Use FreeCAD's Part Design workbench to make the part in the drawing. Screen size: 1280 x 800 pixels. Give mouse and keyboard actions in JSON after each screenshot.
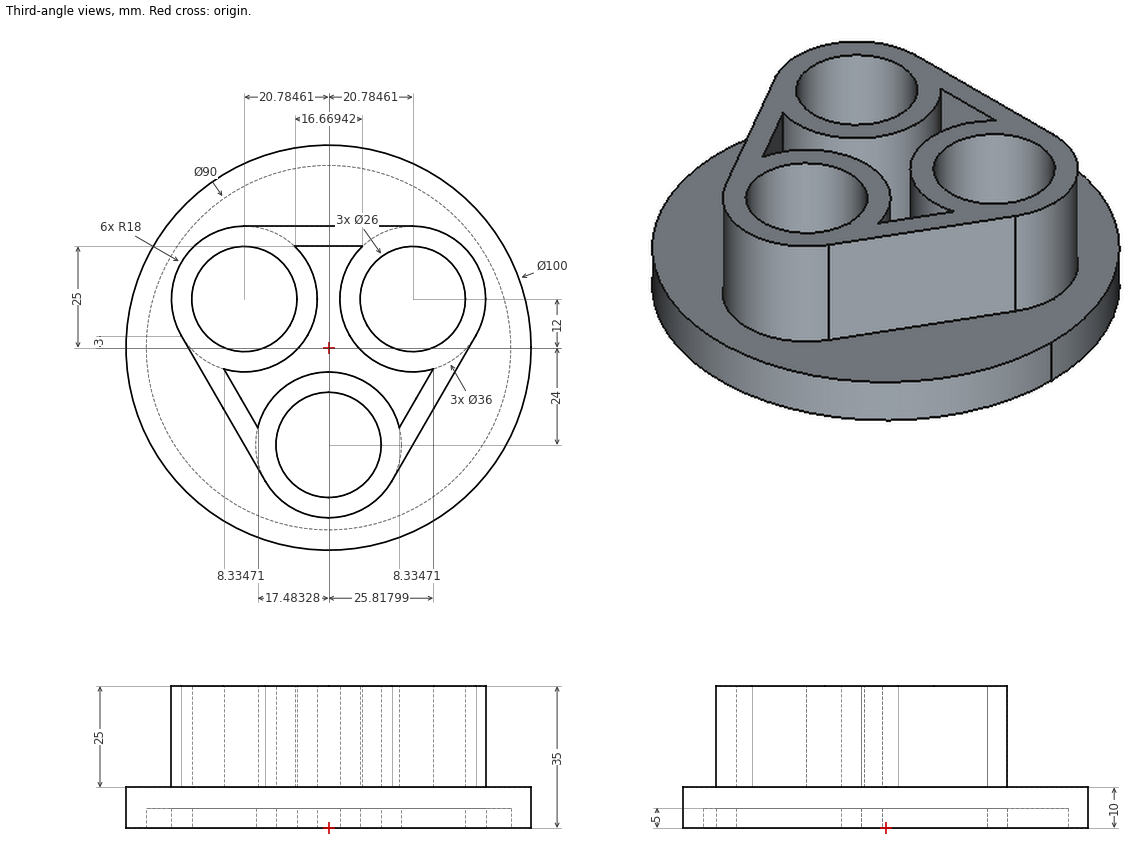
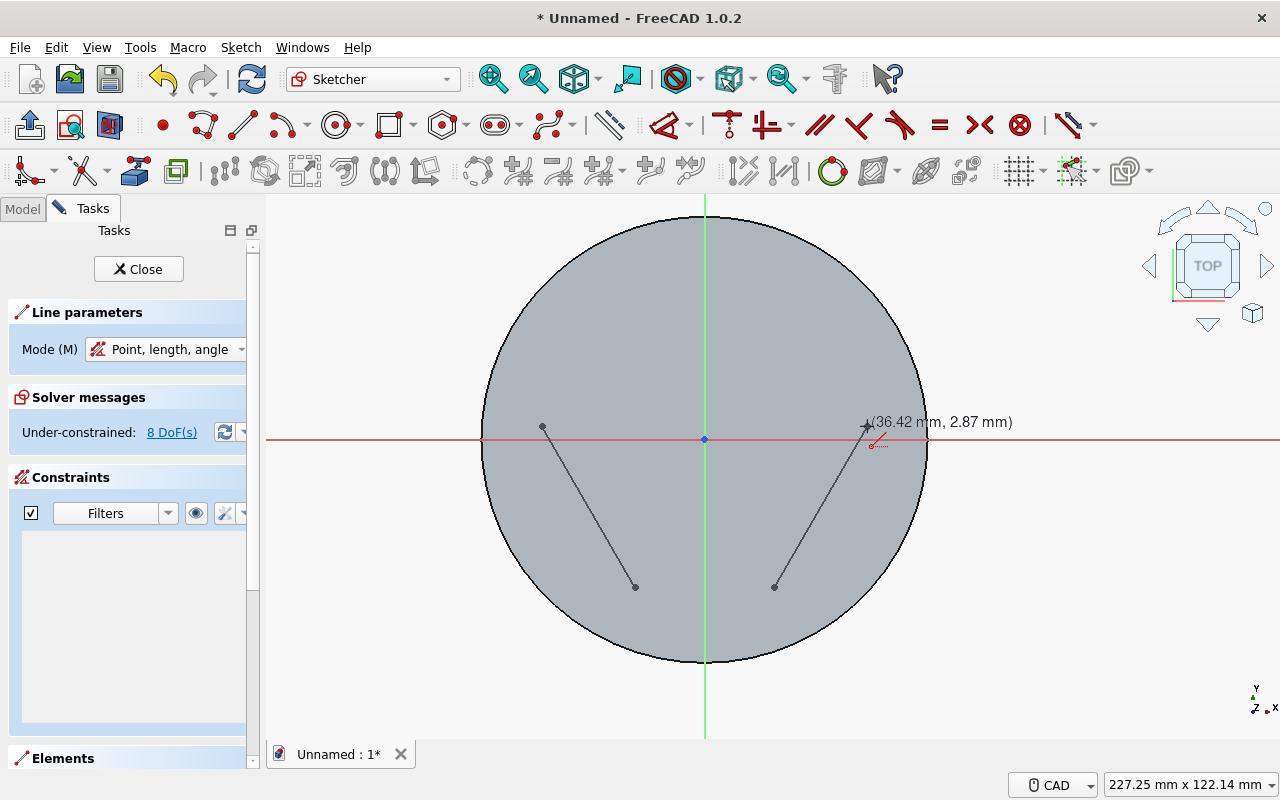
{"action": "left_click", "coordinate": [797, 306]}
{"action": "left_click", "coordinate": [612, 306]}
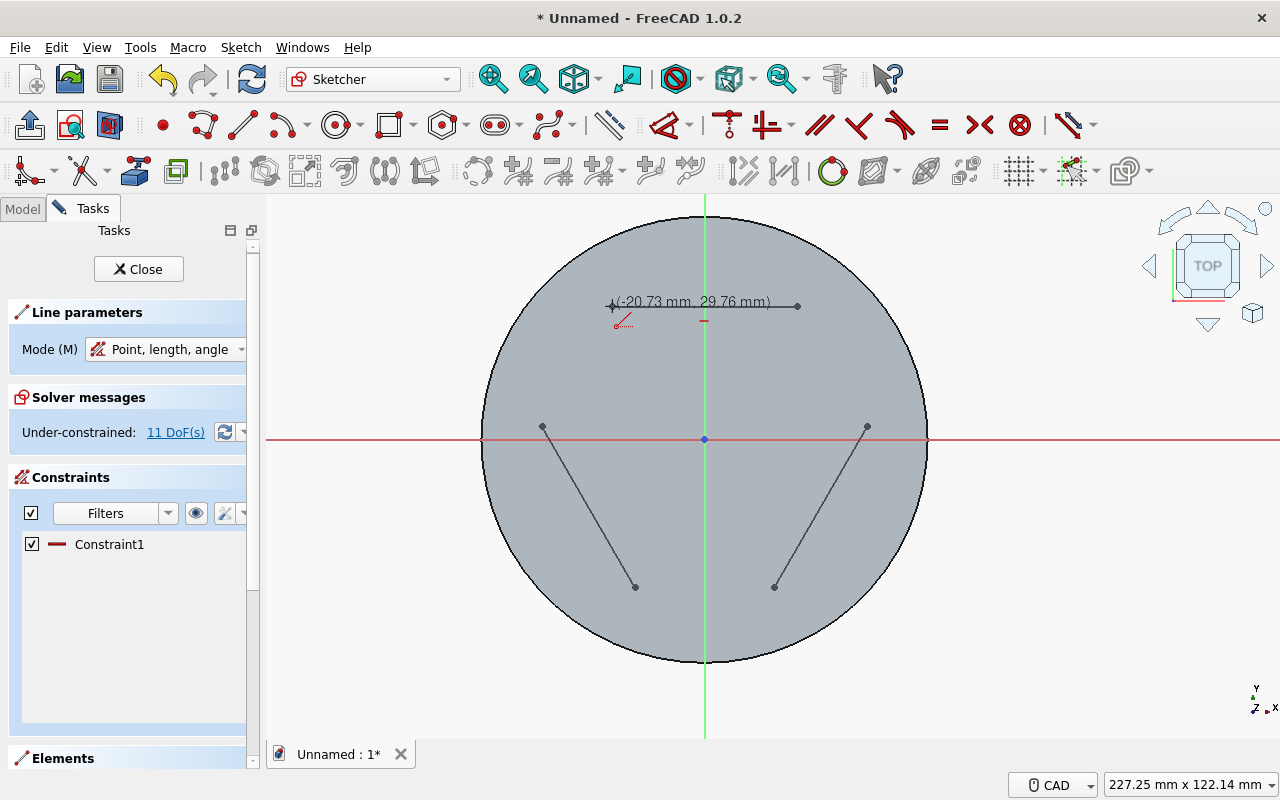
{"action": "left_click", "coordinate": [310, 126]}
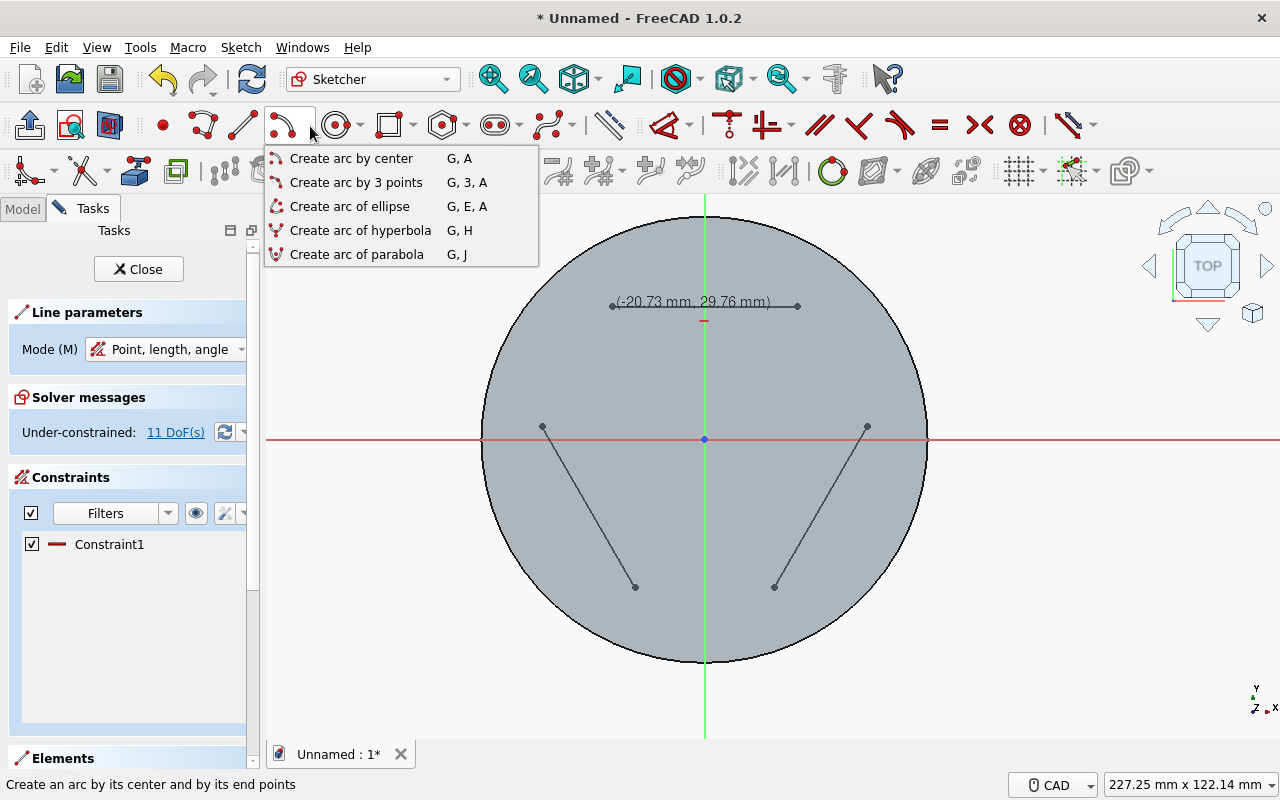
{"action": "left_click", "coordinate": [402, 182]}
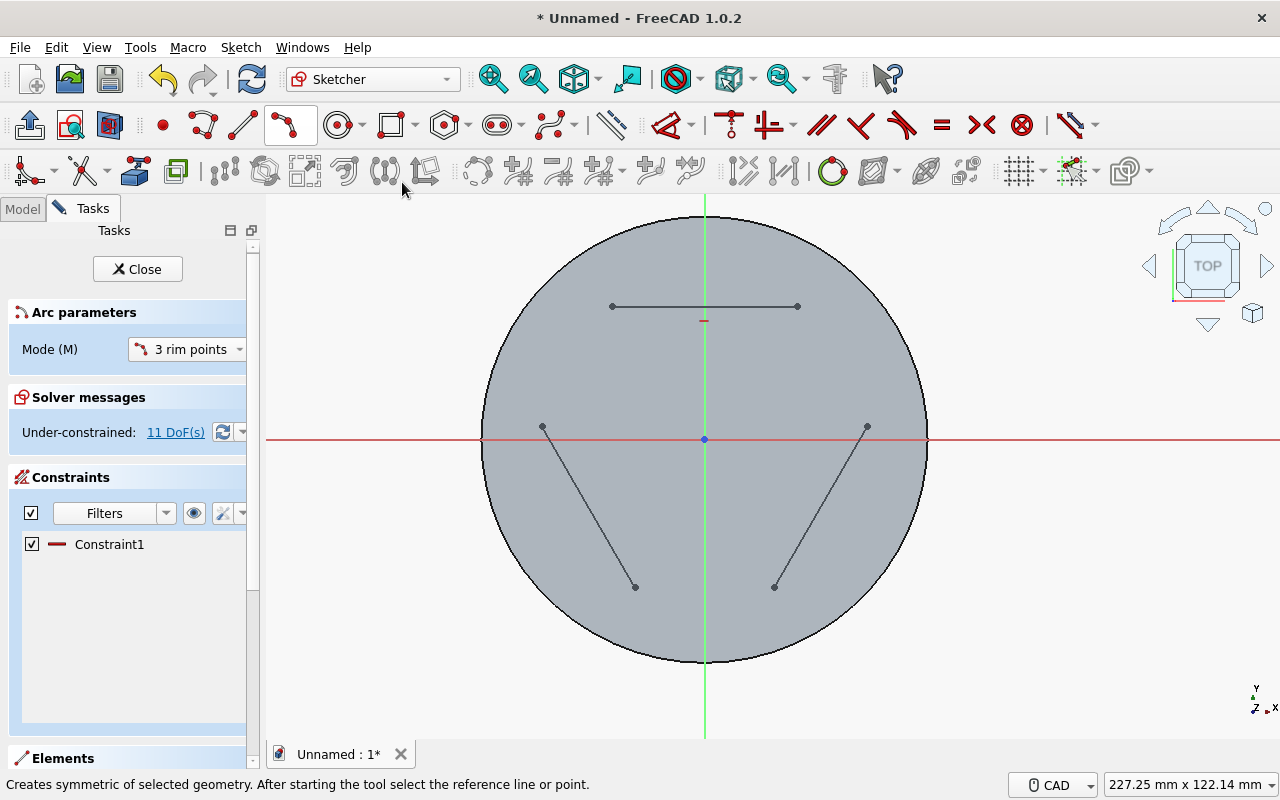
{"action": "left_click", "coordinate": [635, 588]}
{"action": "left_click", "coordinate": [774, 588]}
{"action": "left_click", "coordinate": [688, 625]}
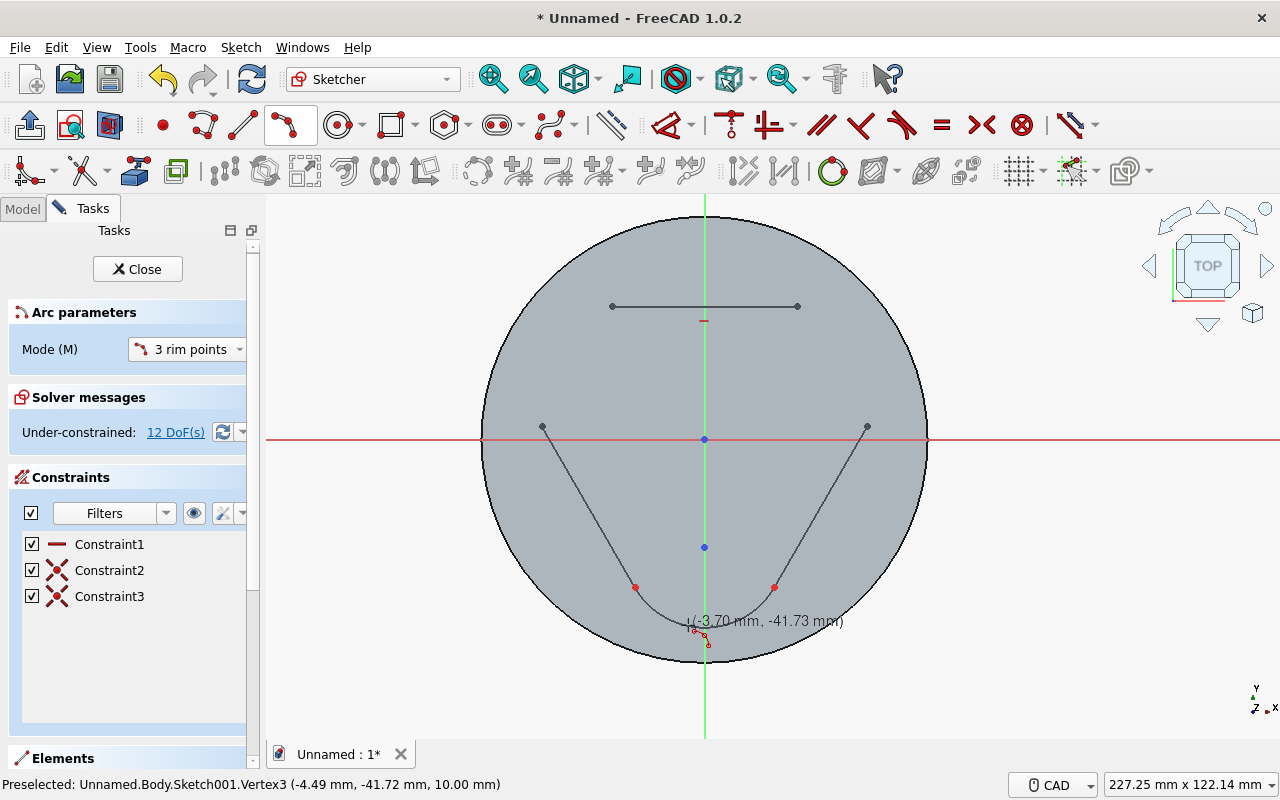
{"action": "left_click", "coordinate": [867, 427]}
{"action": "left_click", "coordinate": [797, 307]}
{"action": "left_click", "coordinate": [867, 346]}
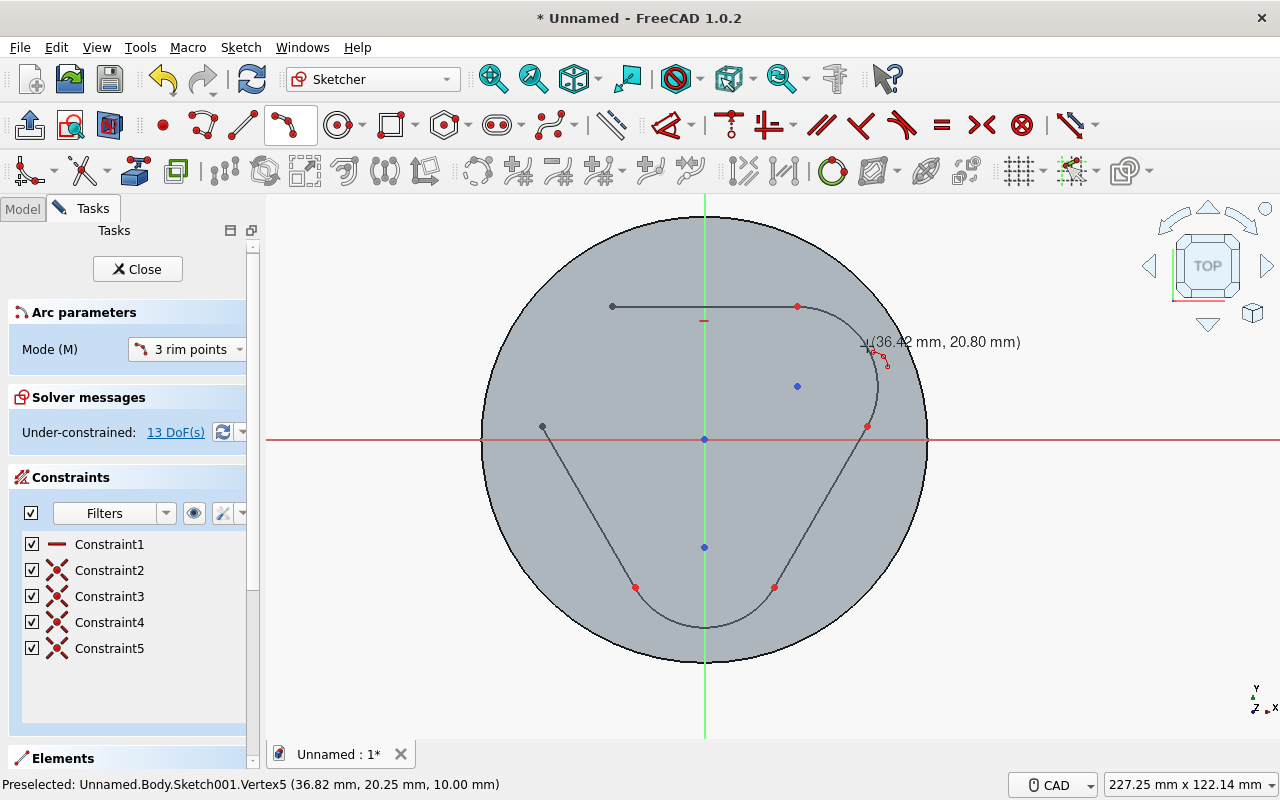
{"action": "left_click", "coordinate": [612, 307]}
{"action": "left_click", "coordinate": [542, 427]}
{"action": "left_click", "coordinate": [542, 346]}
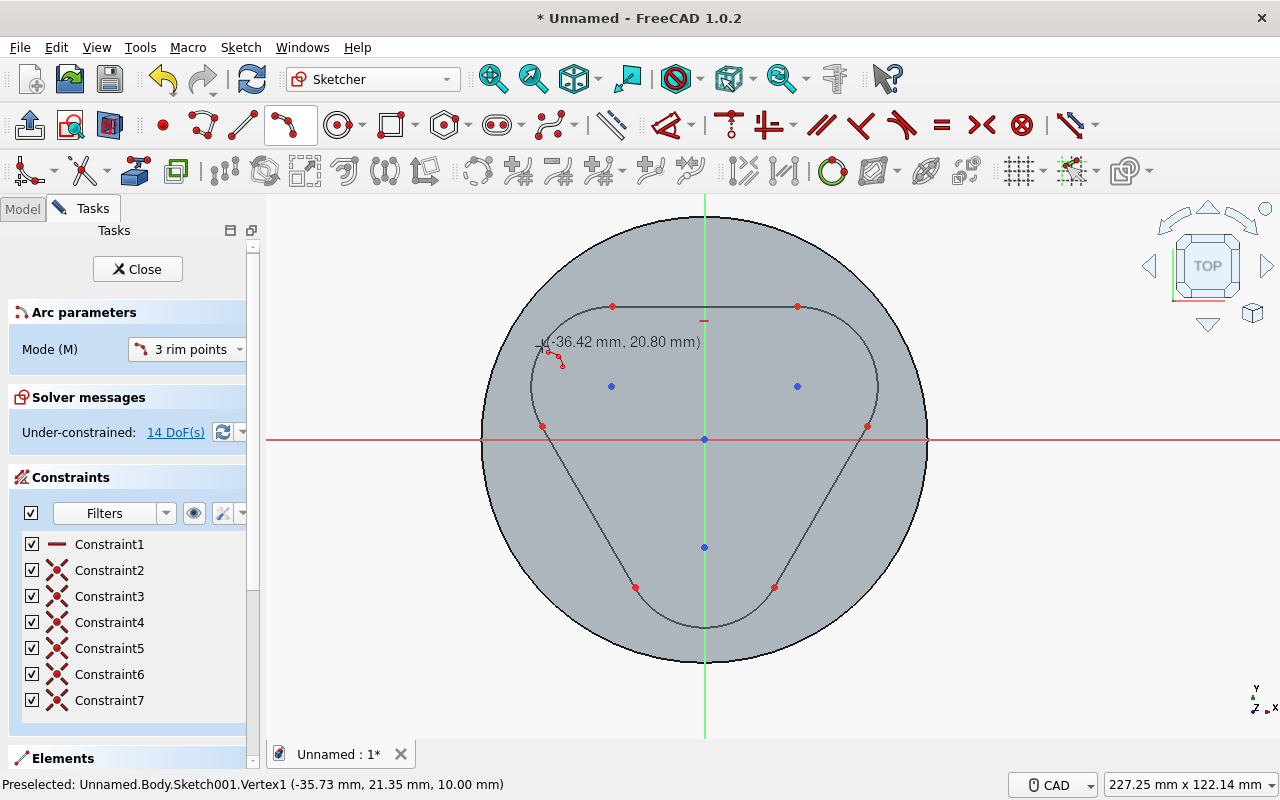
{"action": "left_click", "coordinate": [244, 126]}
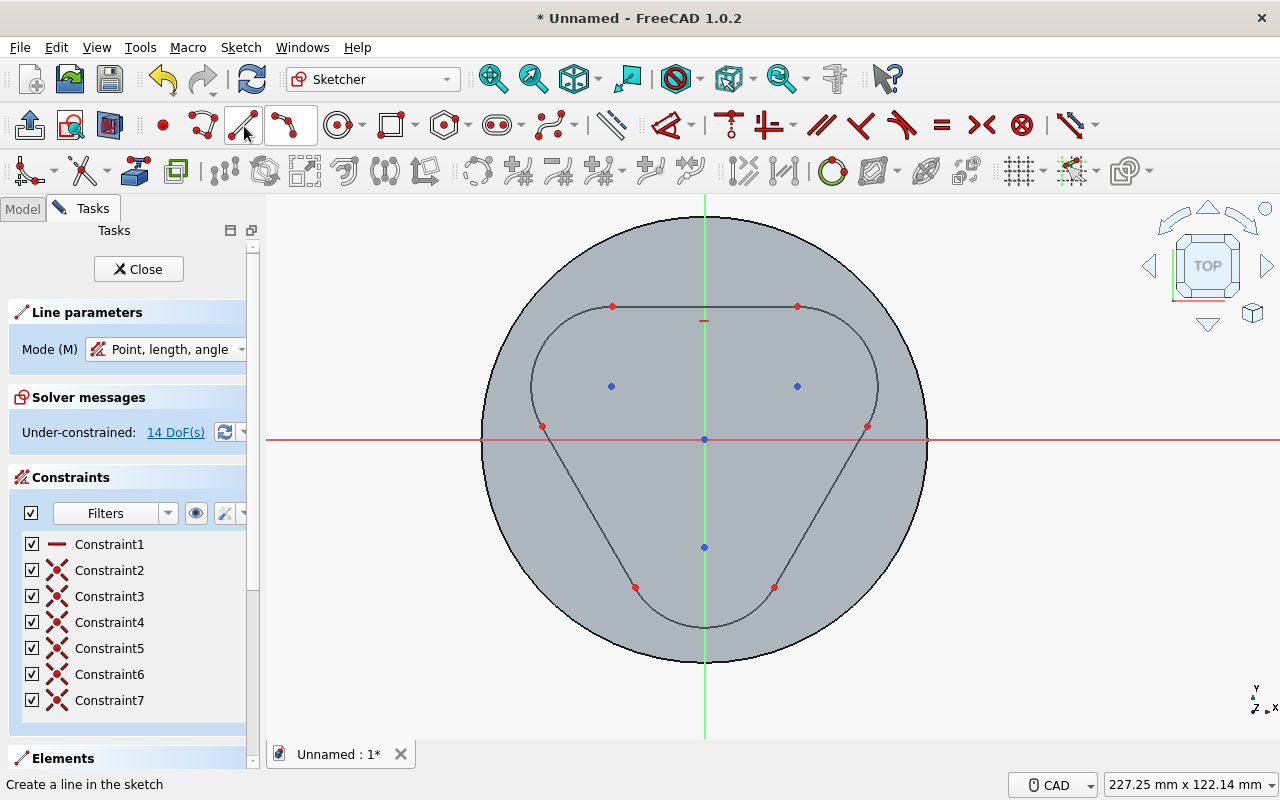
{"action": "left_click", "coordinate": [626, 528]}
{"action": "left_click", "coordinate": [589, 463]}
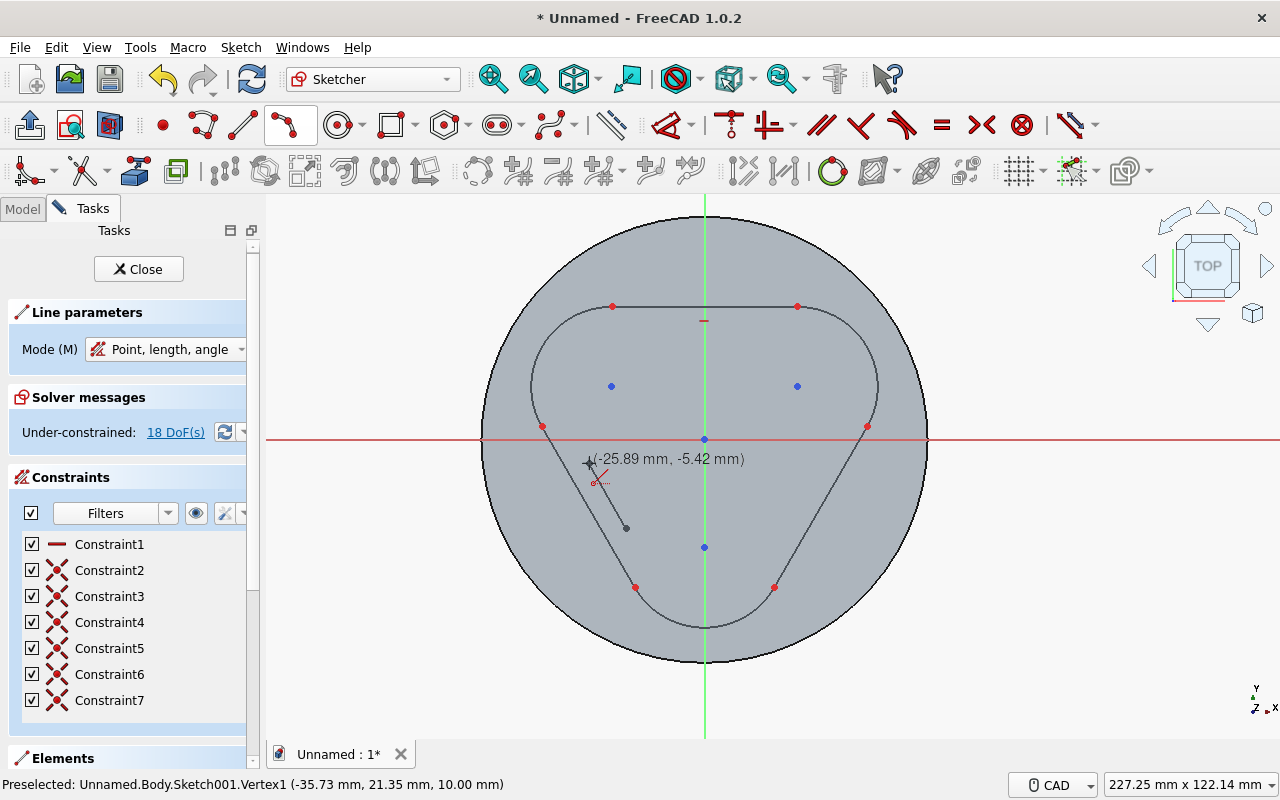
{"action": "left_click", "coordinate": [667, 328]}
{"action": "left_click", "coordinate": [742, 328]}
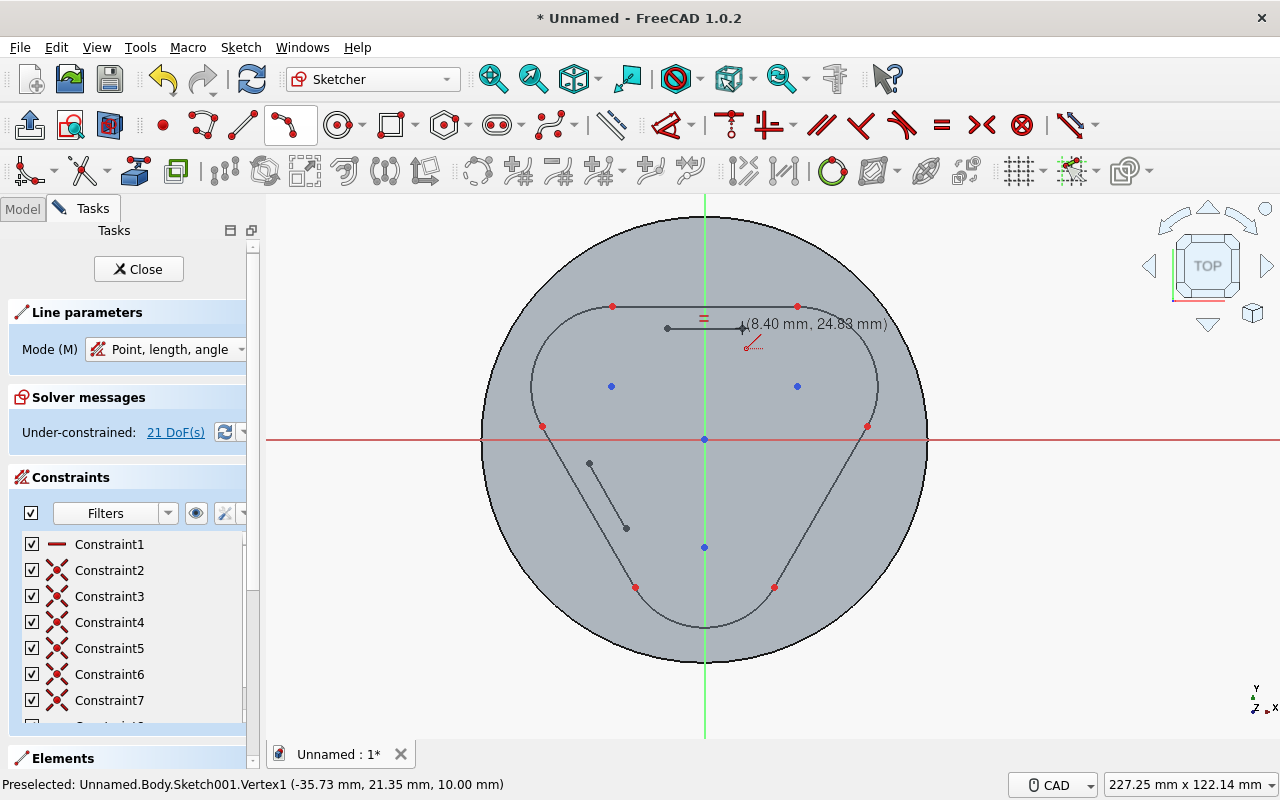
{"action": "left_click", "coordinate": [820, 463]}
{"action": "left_click", "coordinate": [783, 528]}